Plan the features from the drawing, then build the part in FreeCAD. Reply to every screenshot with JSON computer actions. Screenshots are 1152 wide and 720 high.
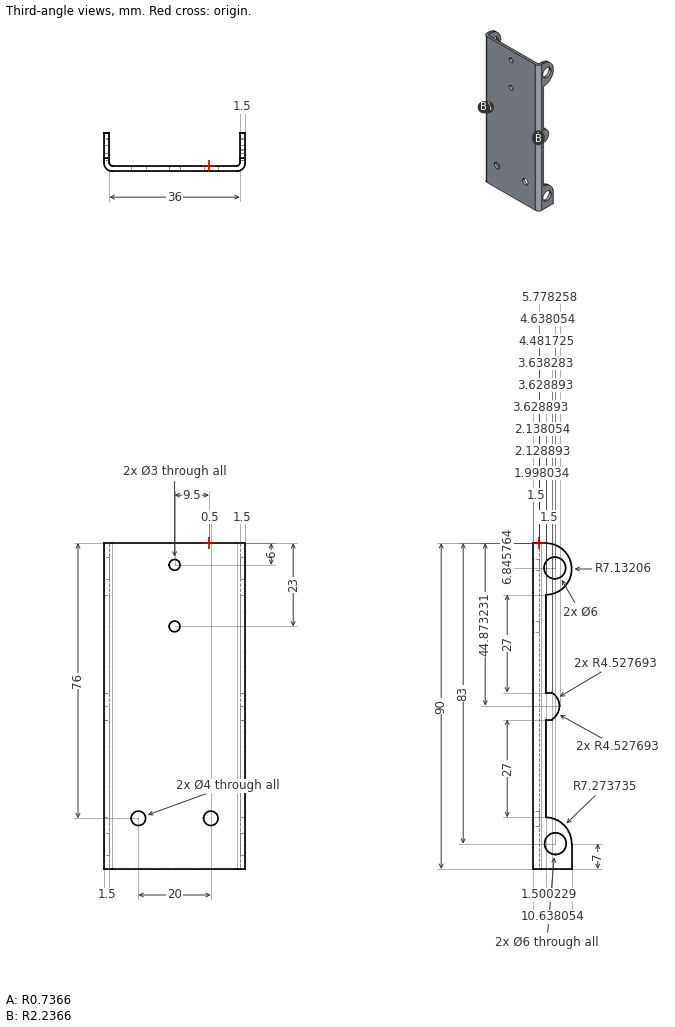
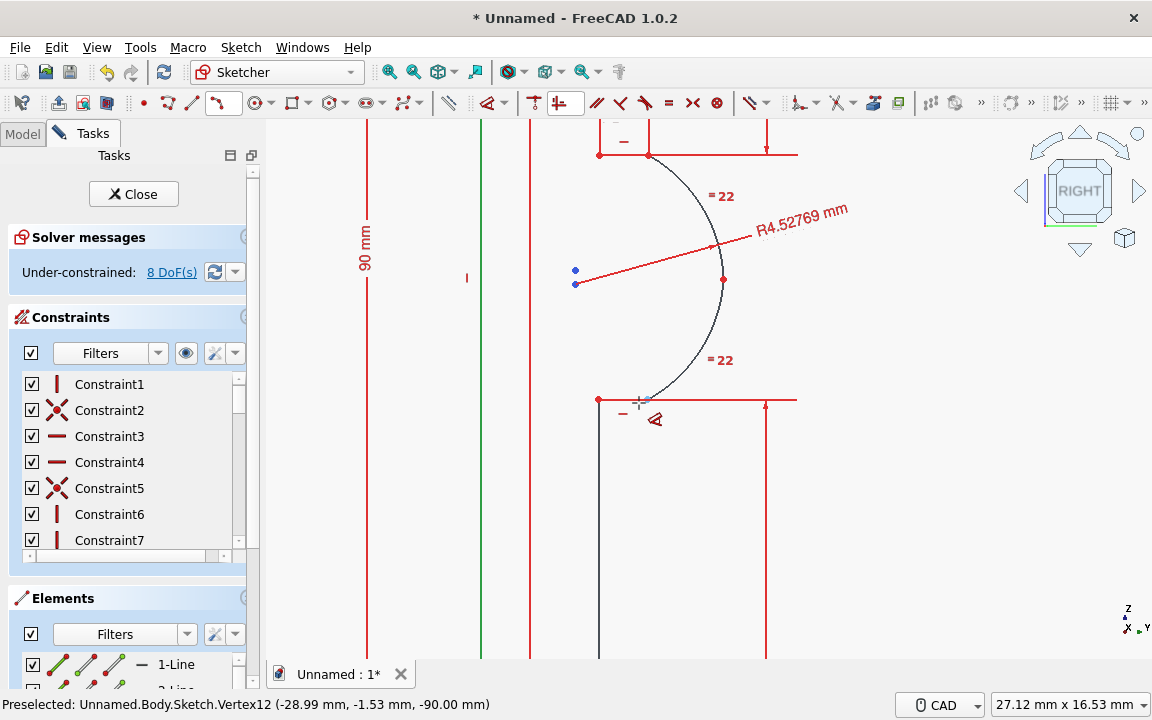
{"action": "left_click", "coordinate": [633, 400]}
{"action": "left_click", "coordinate": [623, 434]}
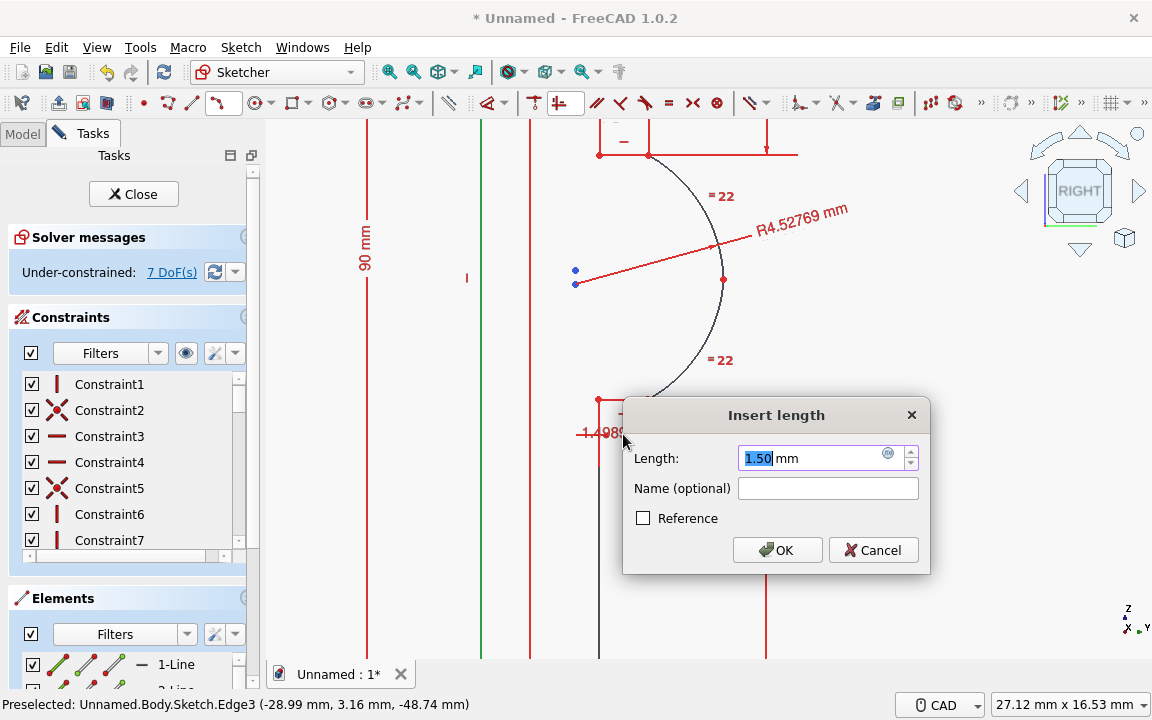
{"action": "type", "text": "1.500229"}
{"action": "key", "text": "Return"}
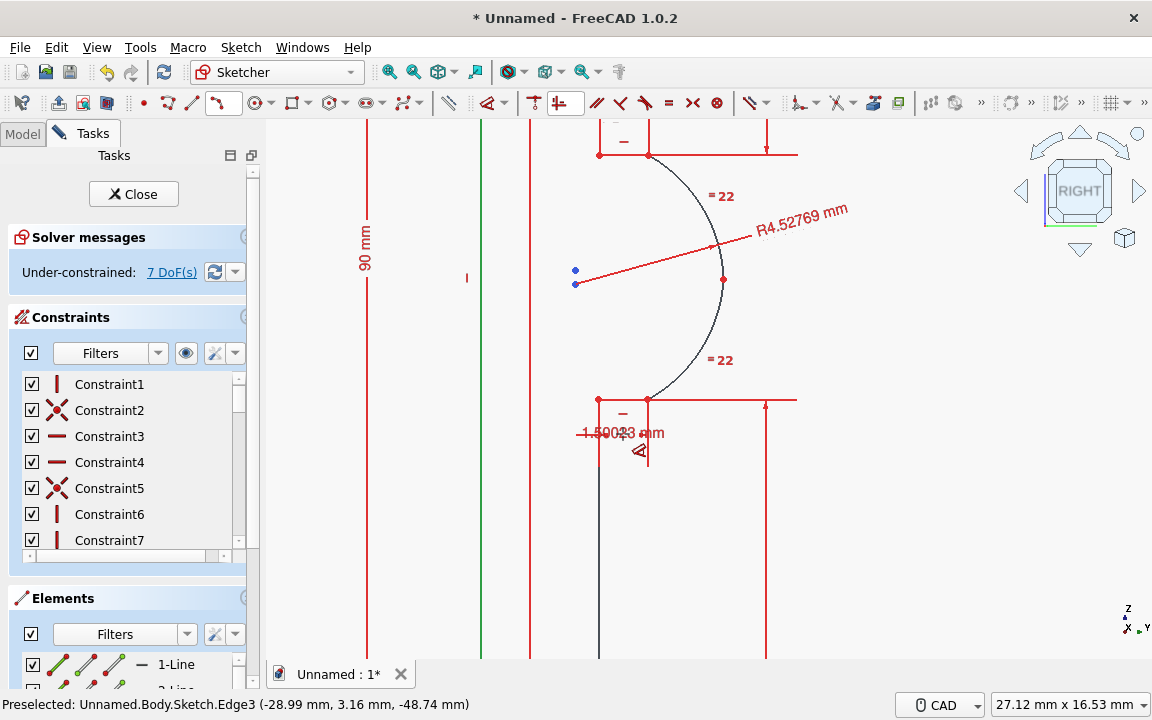
{"action": "scroll", "coordinate": [639, 403], "scroll_direction": "down", "scroll_amount": 11}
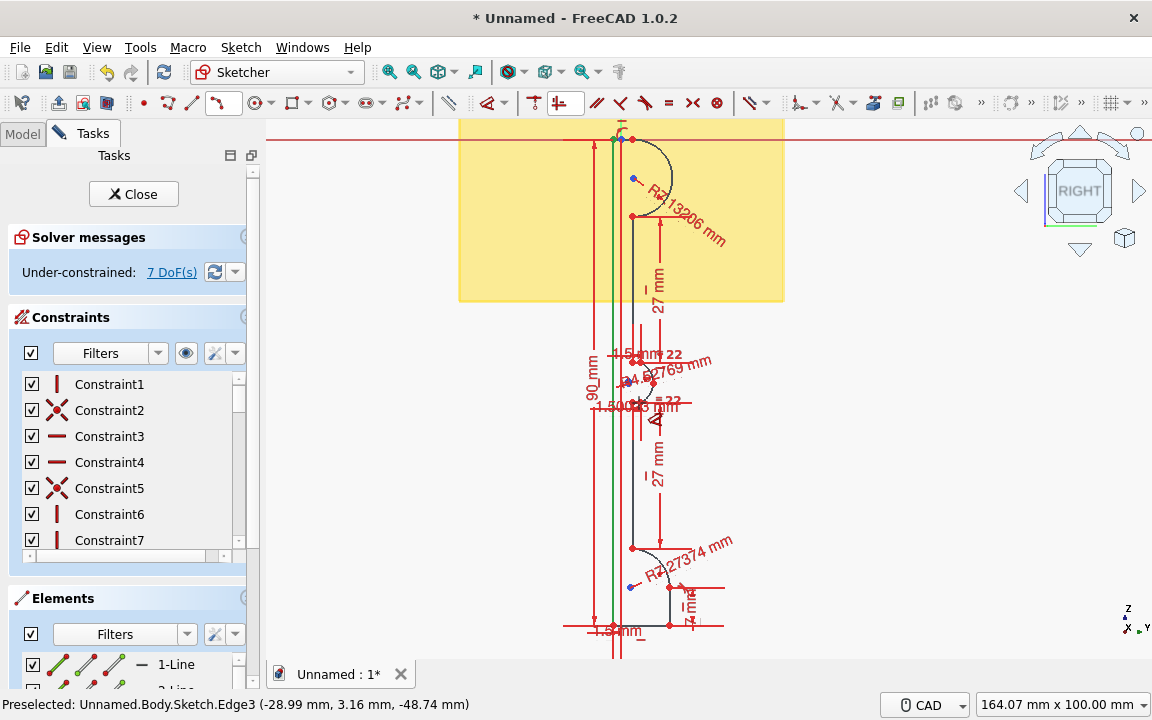
{"action": "scroll", "coordinate": [626, 227], "scroll_direction": "up", "scroll_amount": 12}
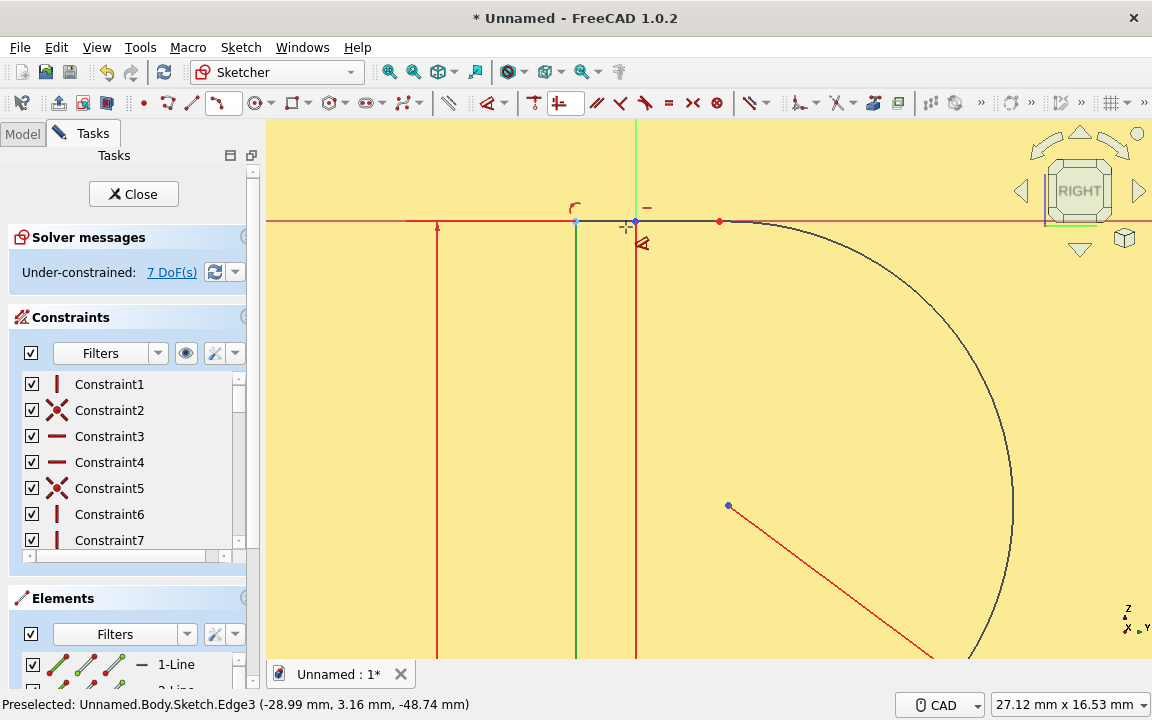
{"action": "left_click", "coordinate": [619, 221]}
{"action": "left_click", "coordinate": [615, 187]}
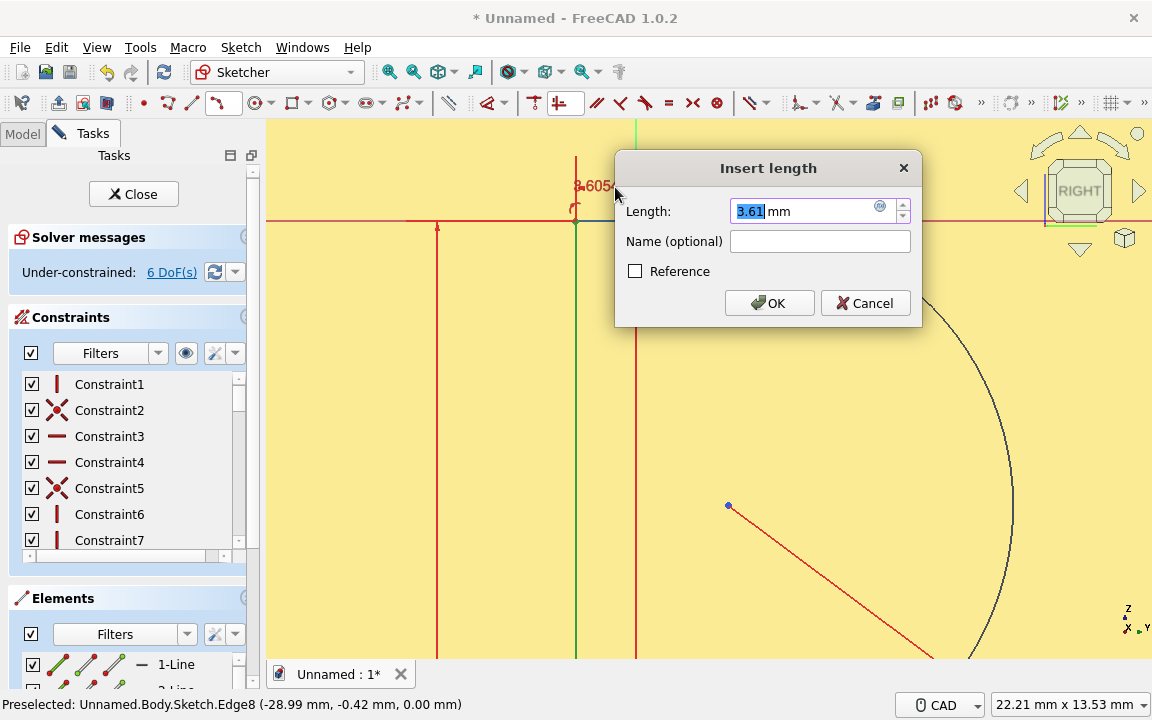
{"action": "type", "text": "3.628893"}
{"action": "key", "text": "Return"}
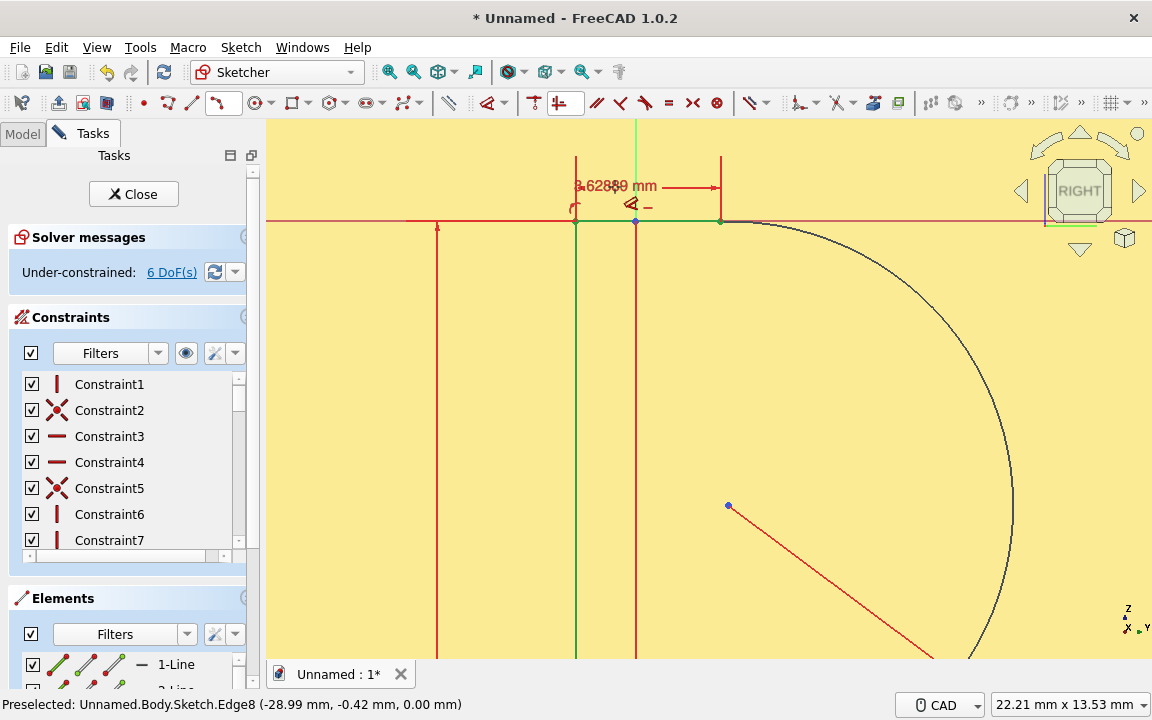
{"action": "scroll", "coordinate": [626, 227], "scroll_direction": "down", "scroll_amount": 12}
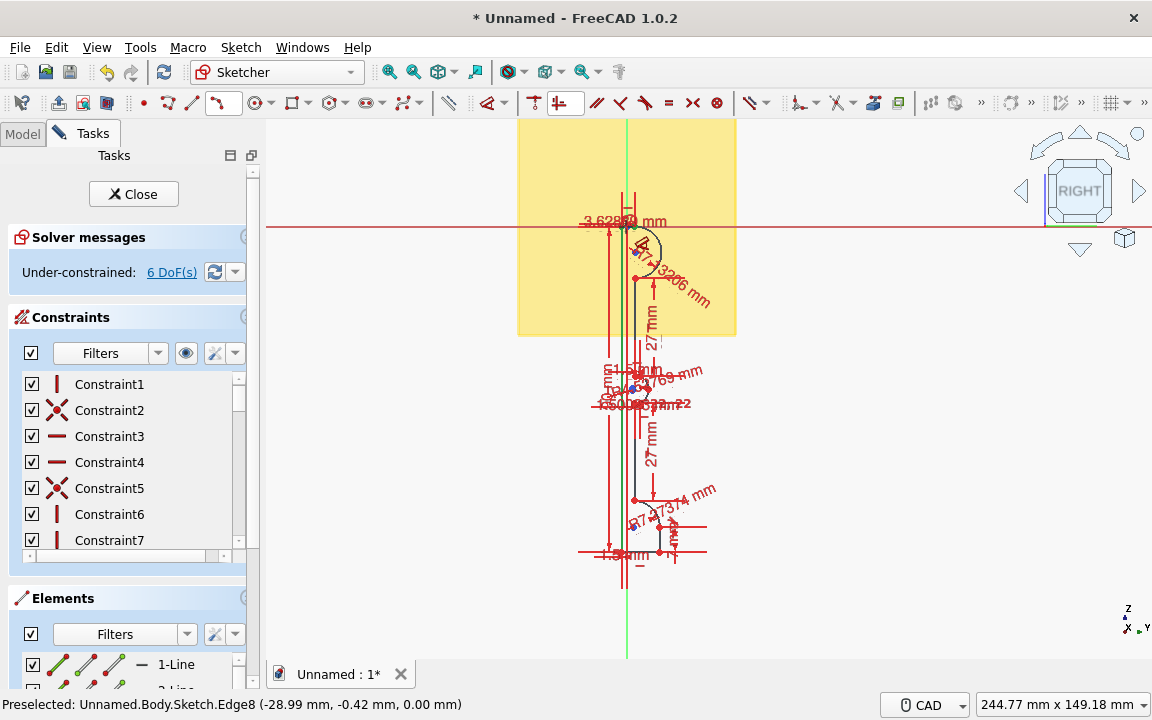
{"action": "left_click", "coordinate": [648, 552]}
{"action": "left_click", "coordinate": [641, 586]}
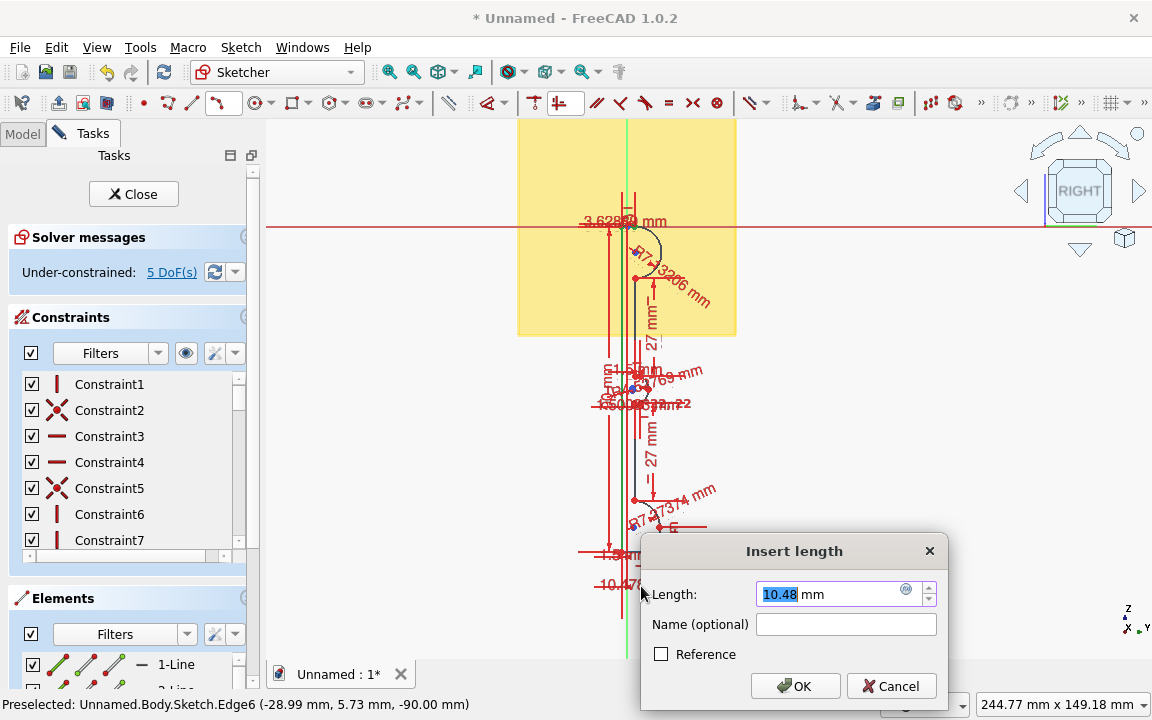
{"action": "type", "text": "10.638054"}
{"action": "key", "text": "Return"}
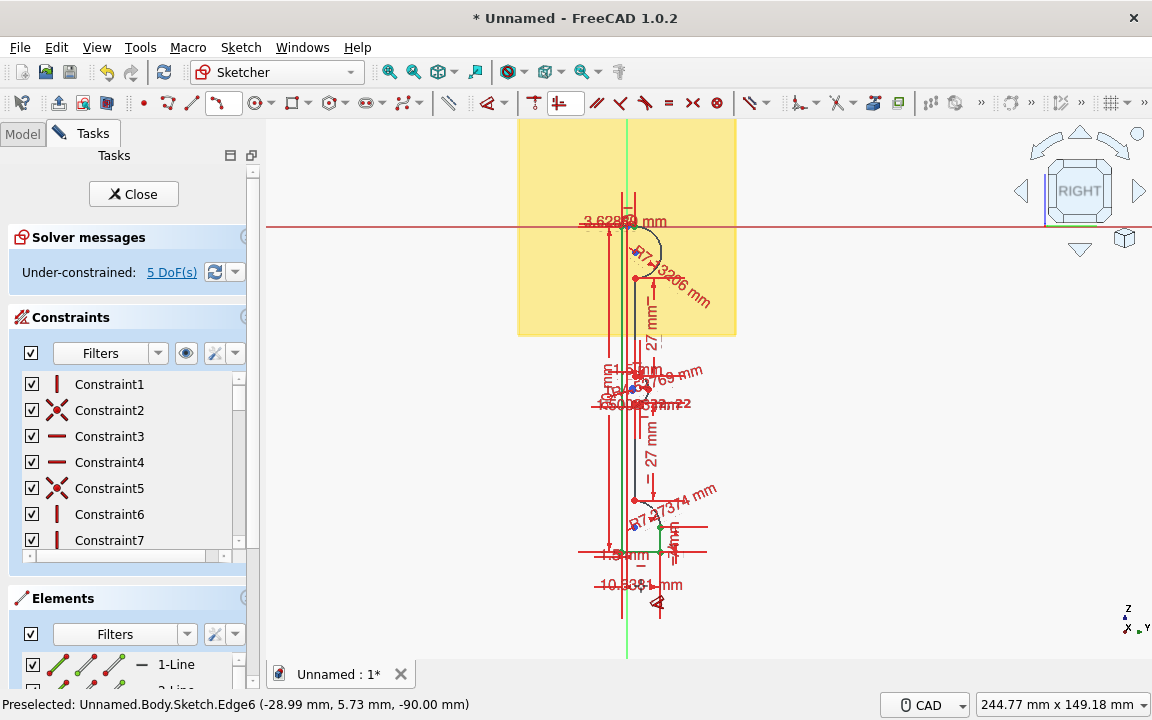
{"action": "scroll", "coordinate": [635, 278], "scroll_direction": "up", "scroll_amount": 9}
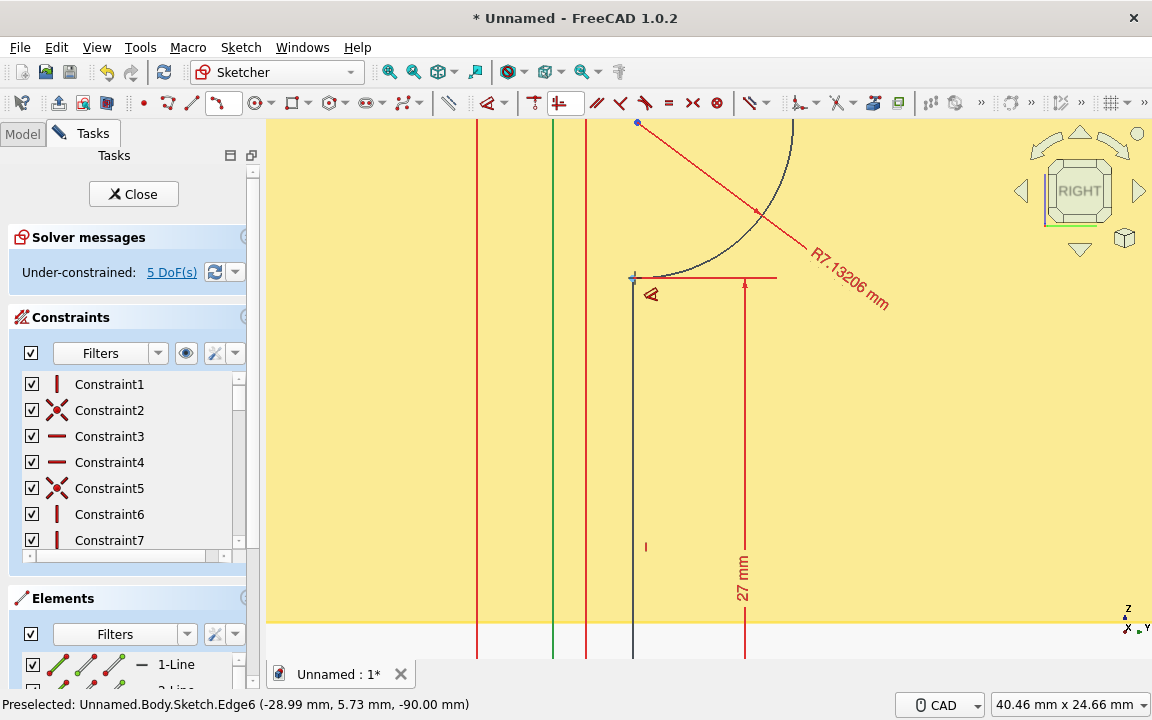
{"action": "left_click", "coordinate": [633, 278]}
{"action": "left_click", "coordinate": [609, 312]}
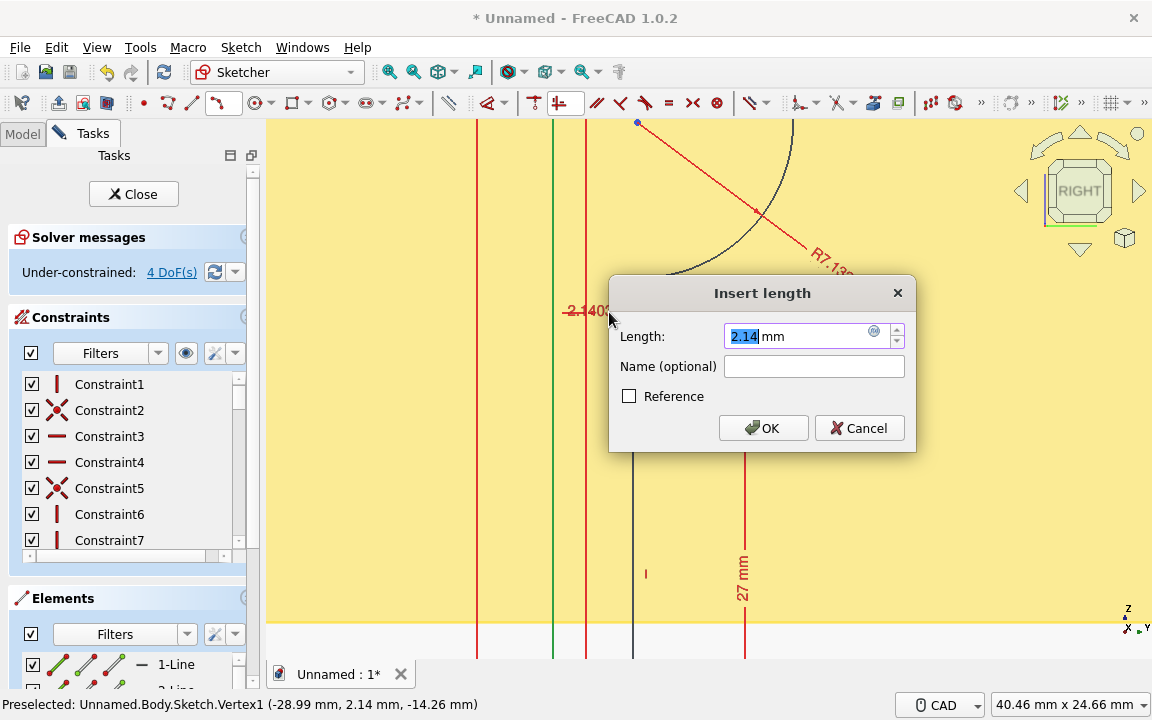
{"action": "type", "text": "2.128893"}
{"action": "key", "text": "Return"}